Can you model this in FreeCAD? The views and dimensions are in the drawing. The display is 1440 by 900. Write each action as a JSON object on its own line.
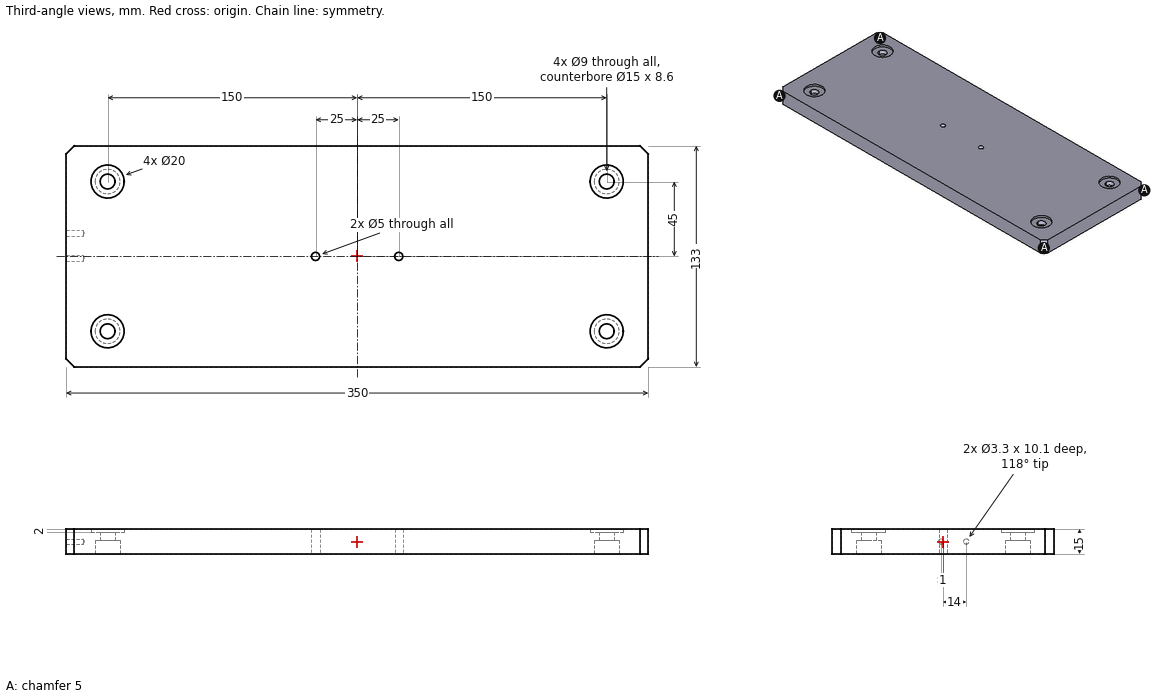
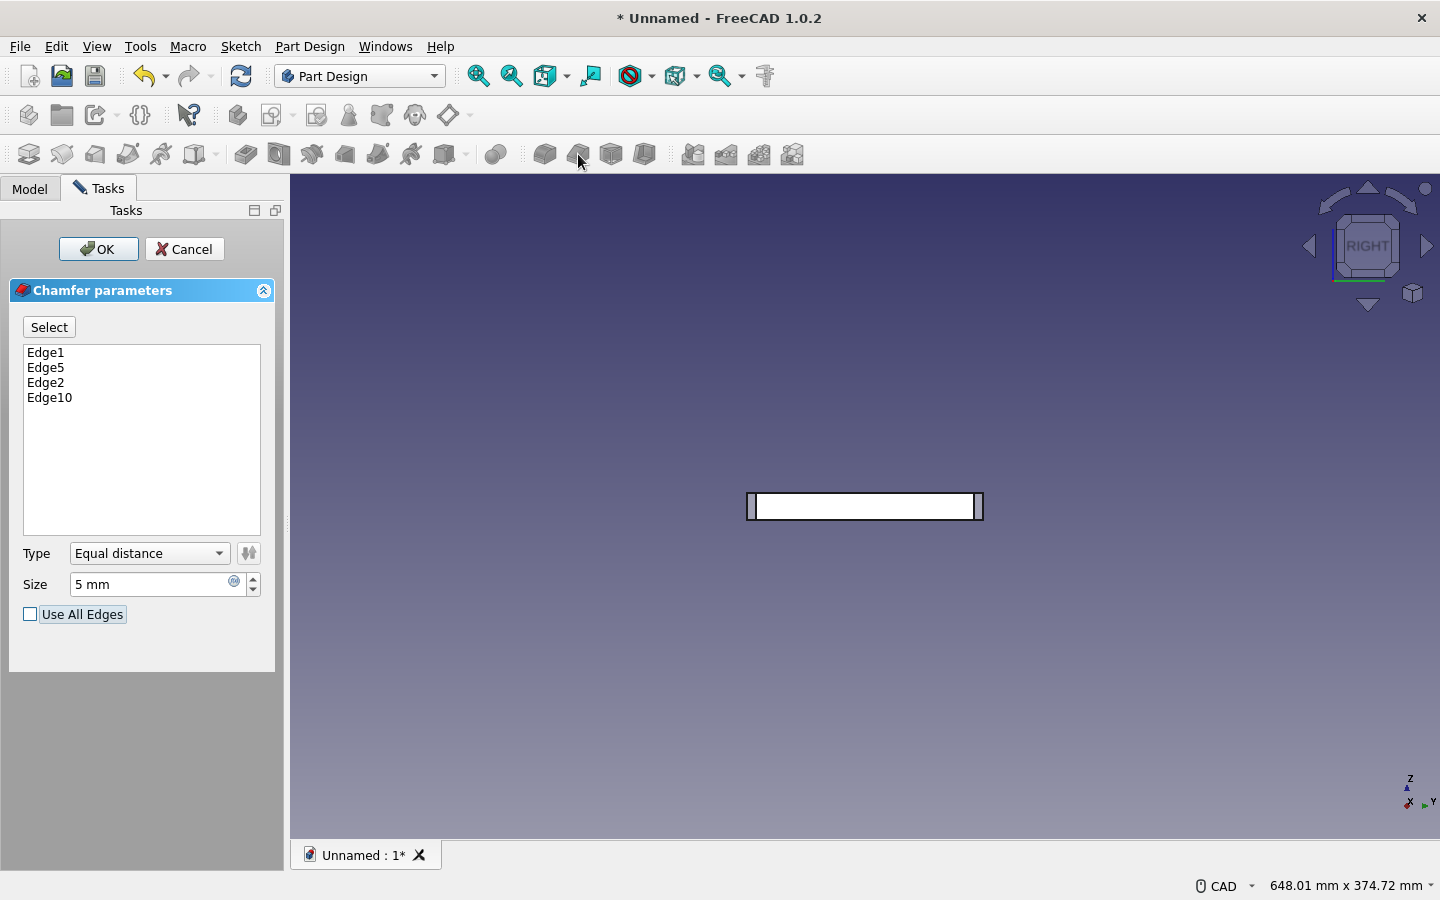
{"action": "left_click", "coordinate": [99, 249]}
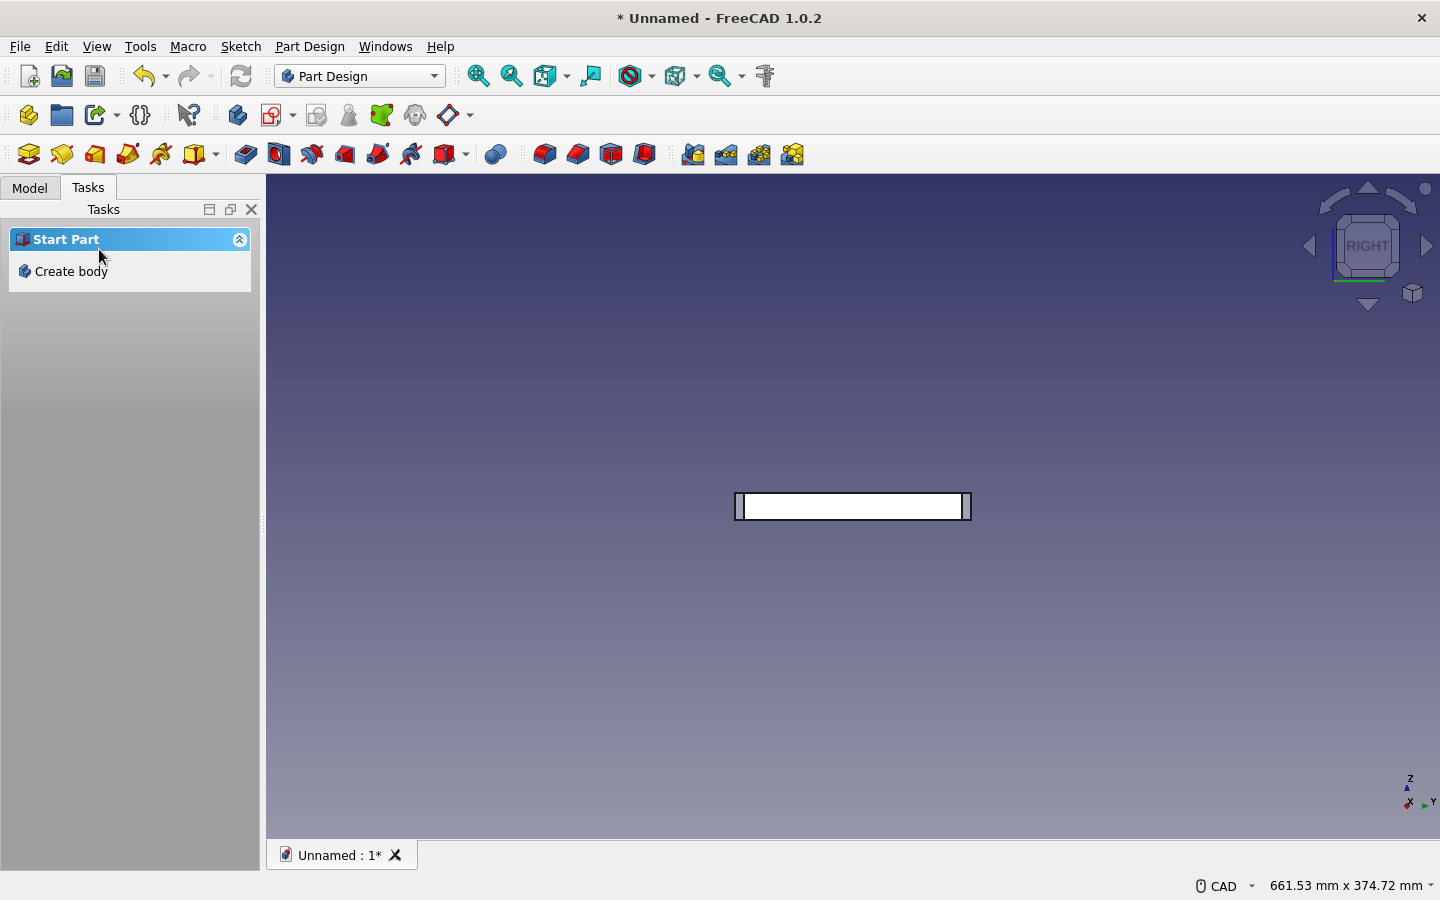
{"action": "key", "text": "0"}